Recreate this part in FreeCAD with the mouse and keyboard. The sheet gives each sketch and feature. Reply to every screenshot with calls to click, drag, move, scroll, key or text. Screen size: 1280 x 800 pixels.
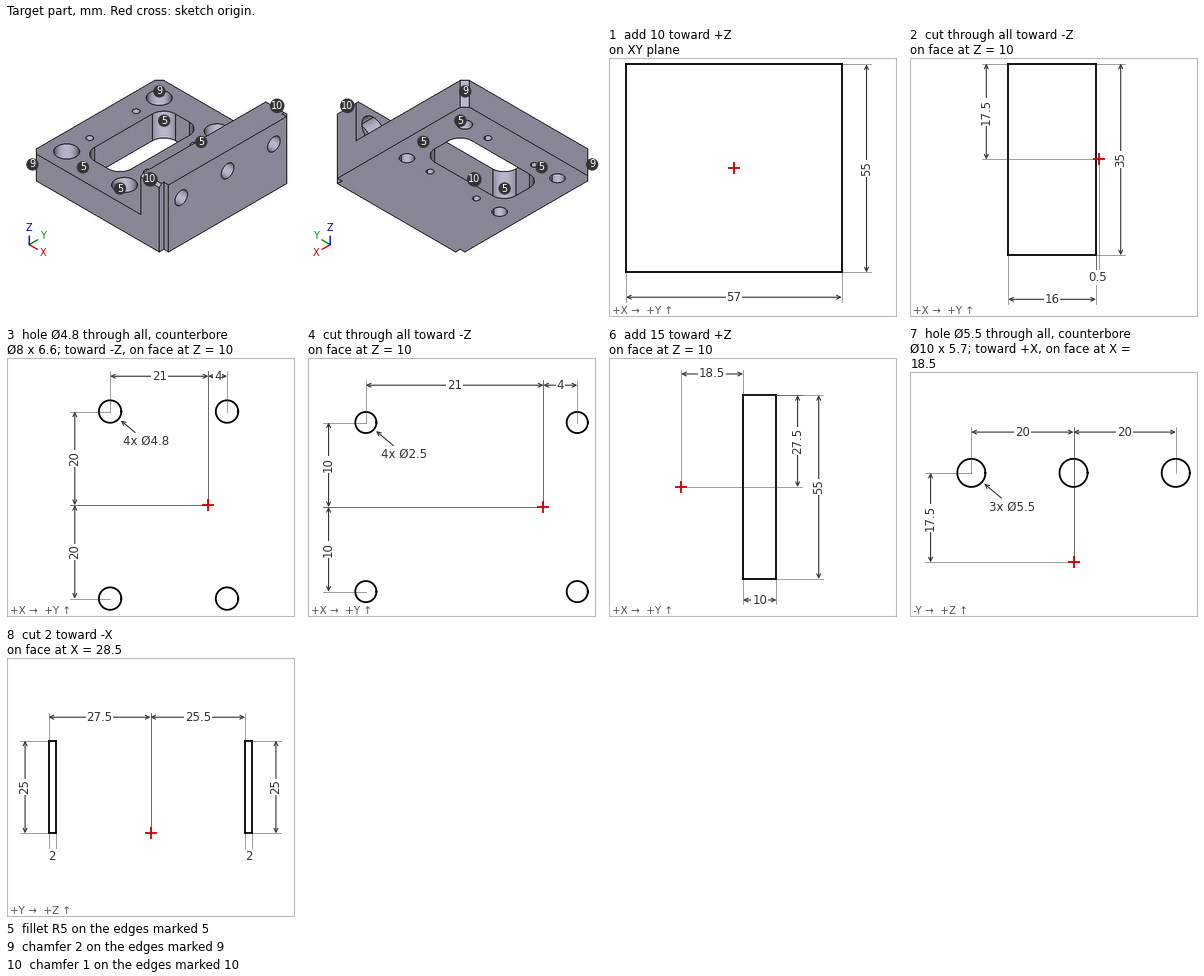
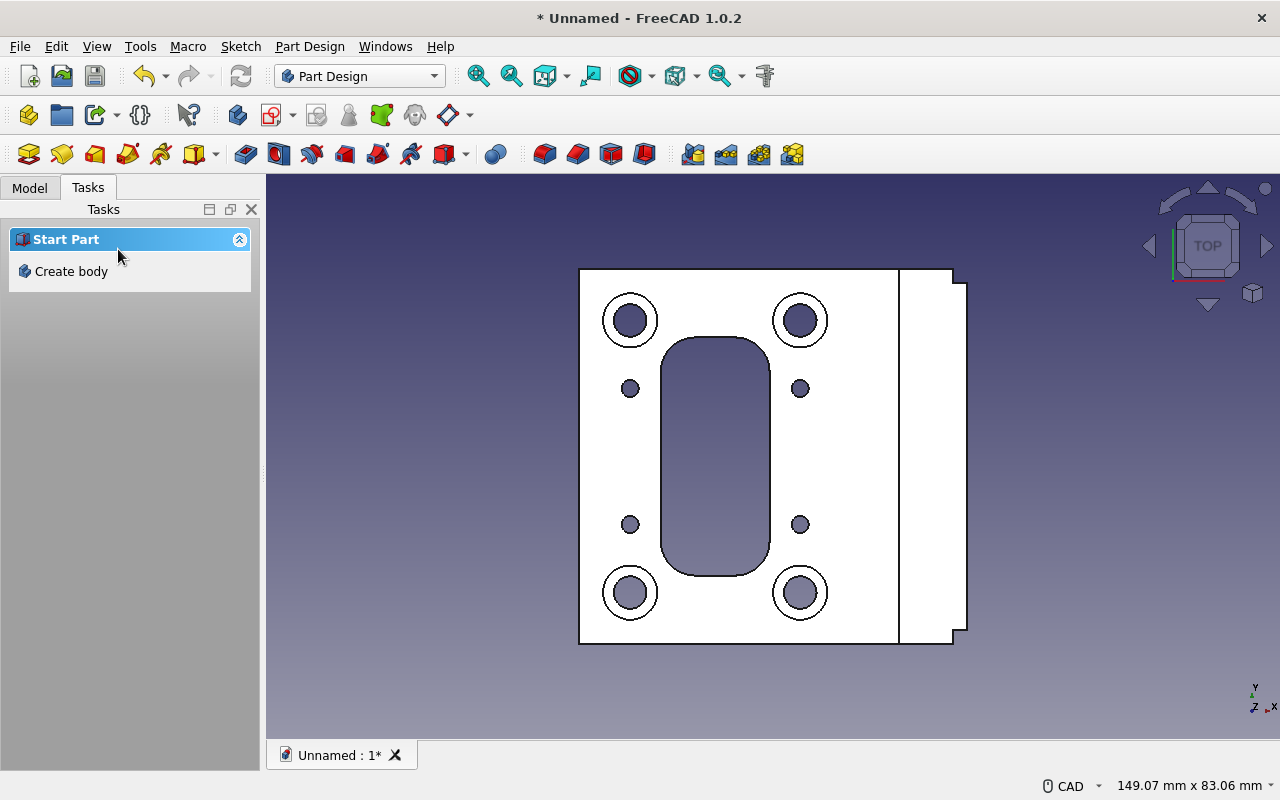
key(0)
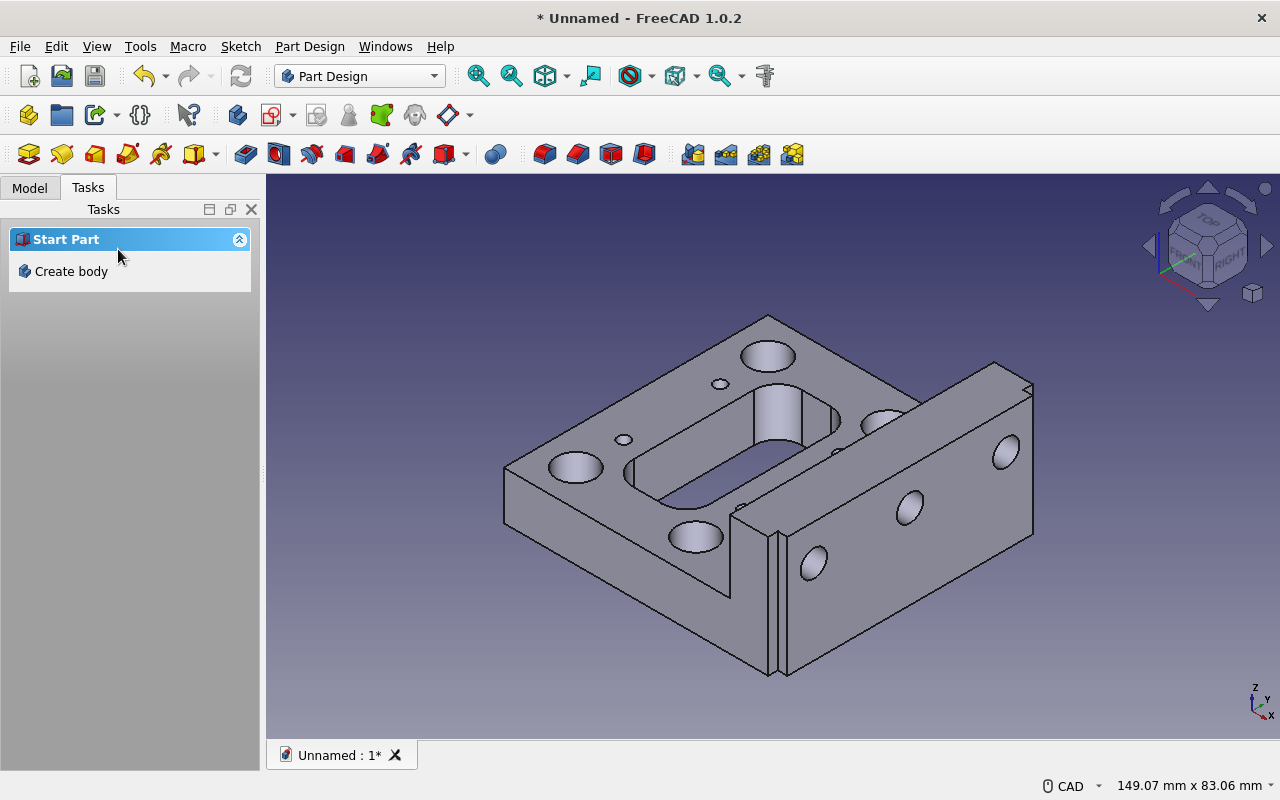
key(1)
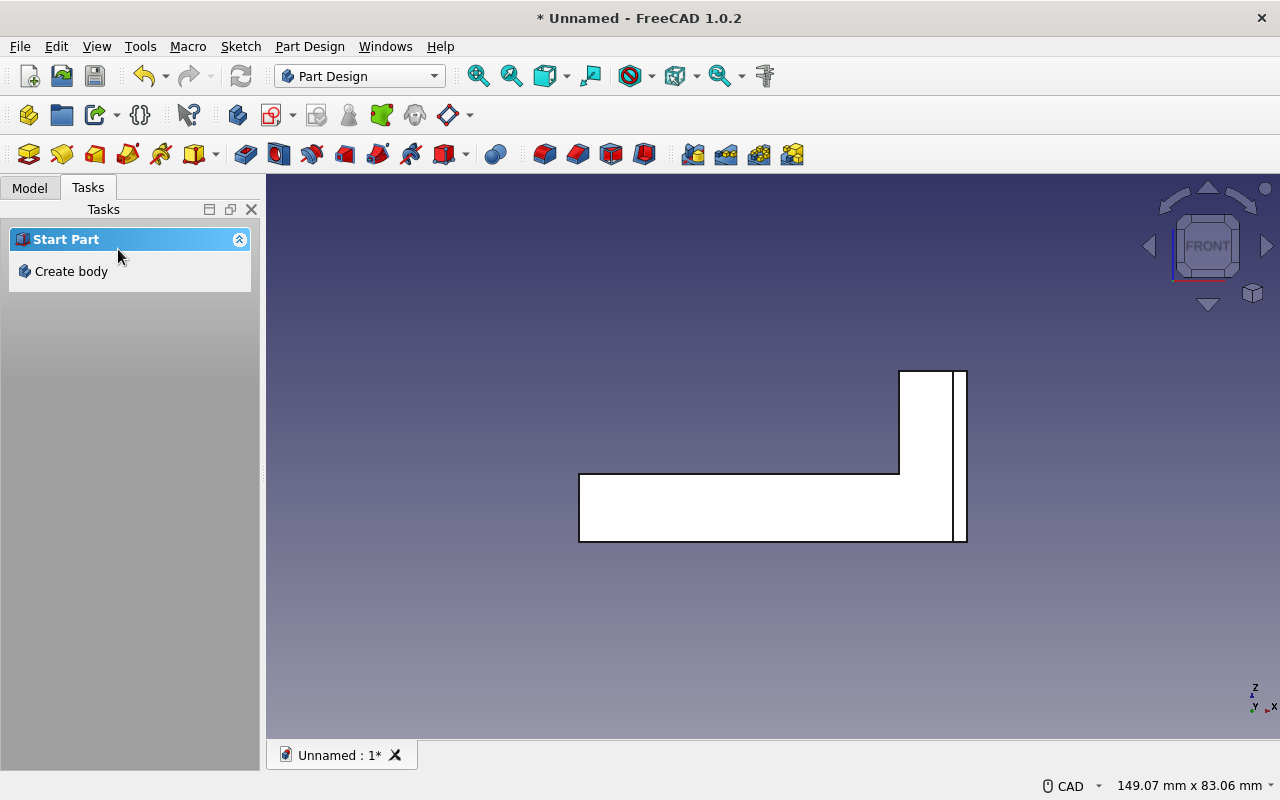
click(479, 76)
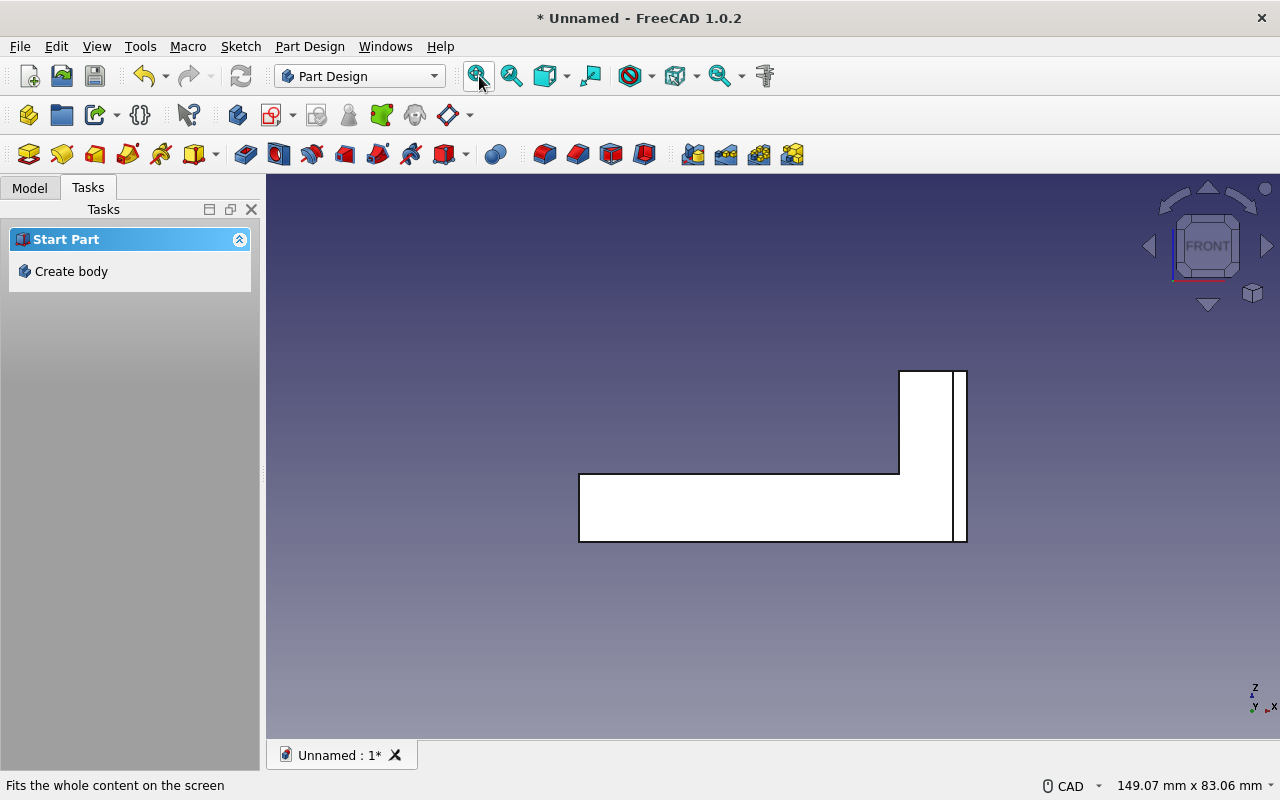
click(579, 507)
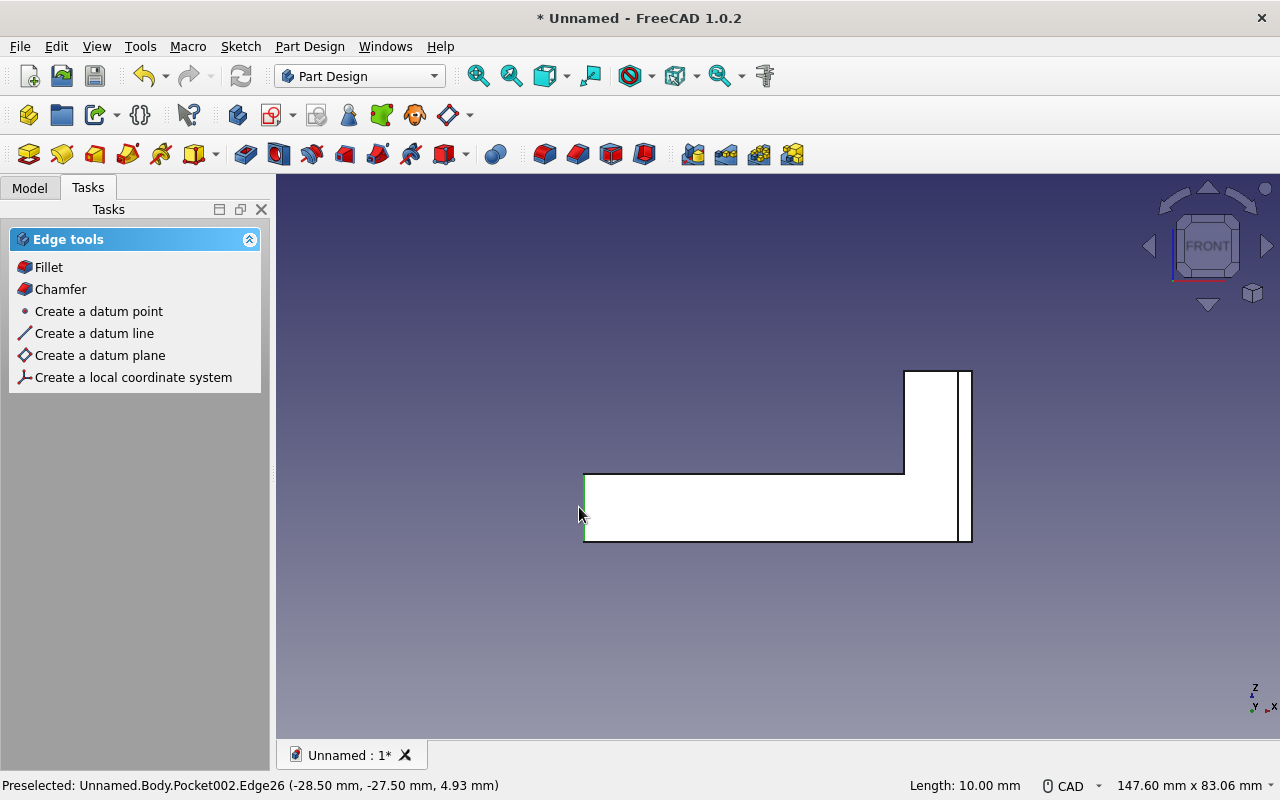
key(3)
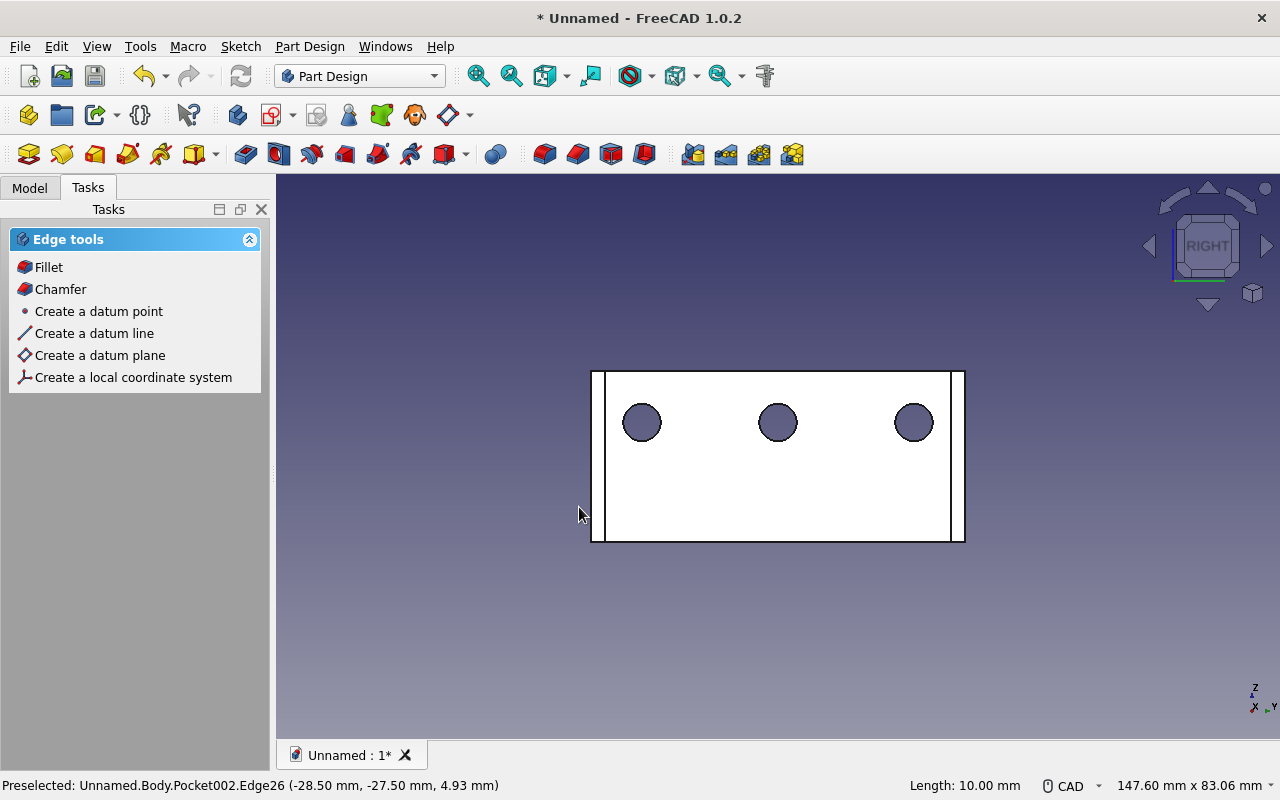
click(479, 76)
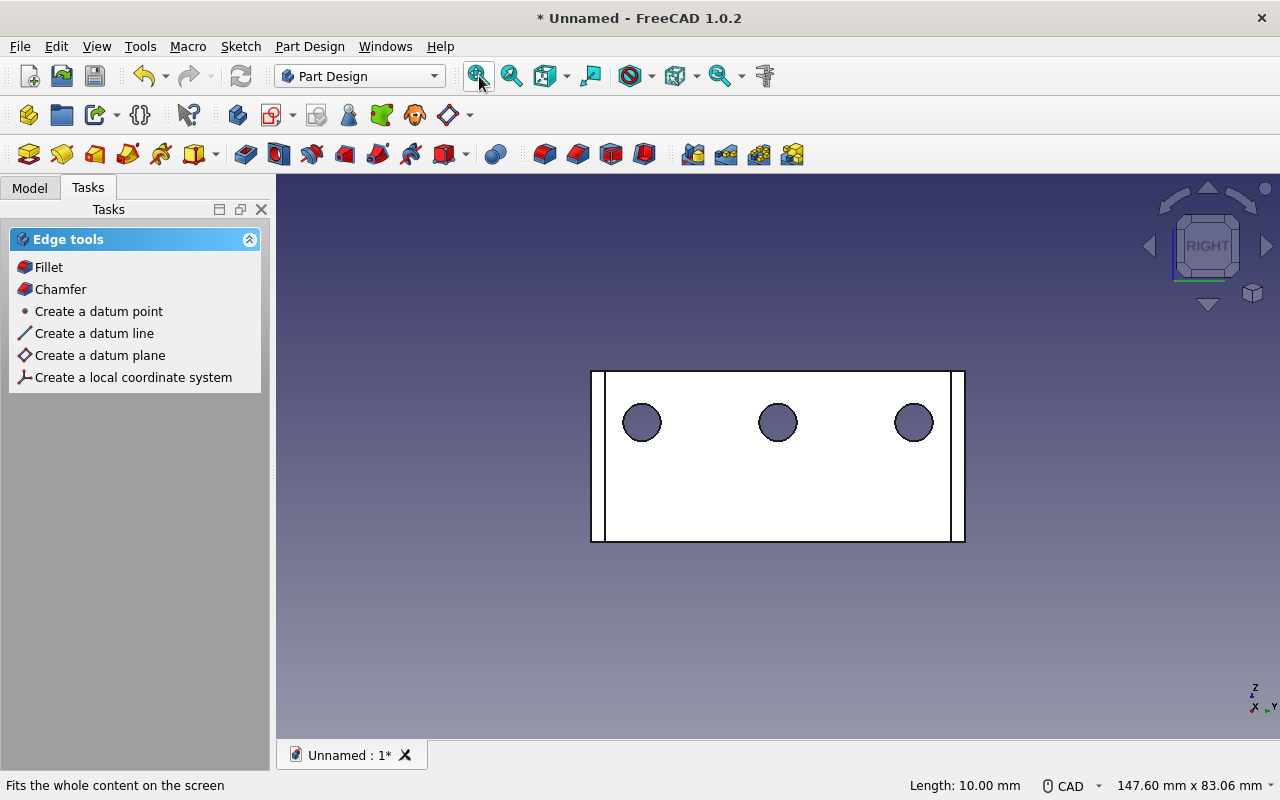
key(5)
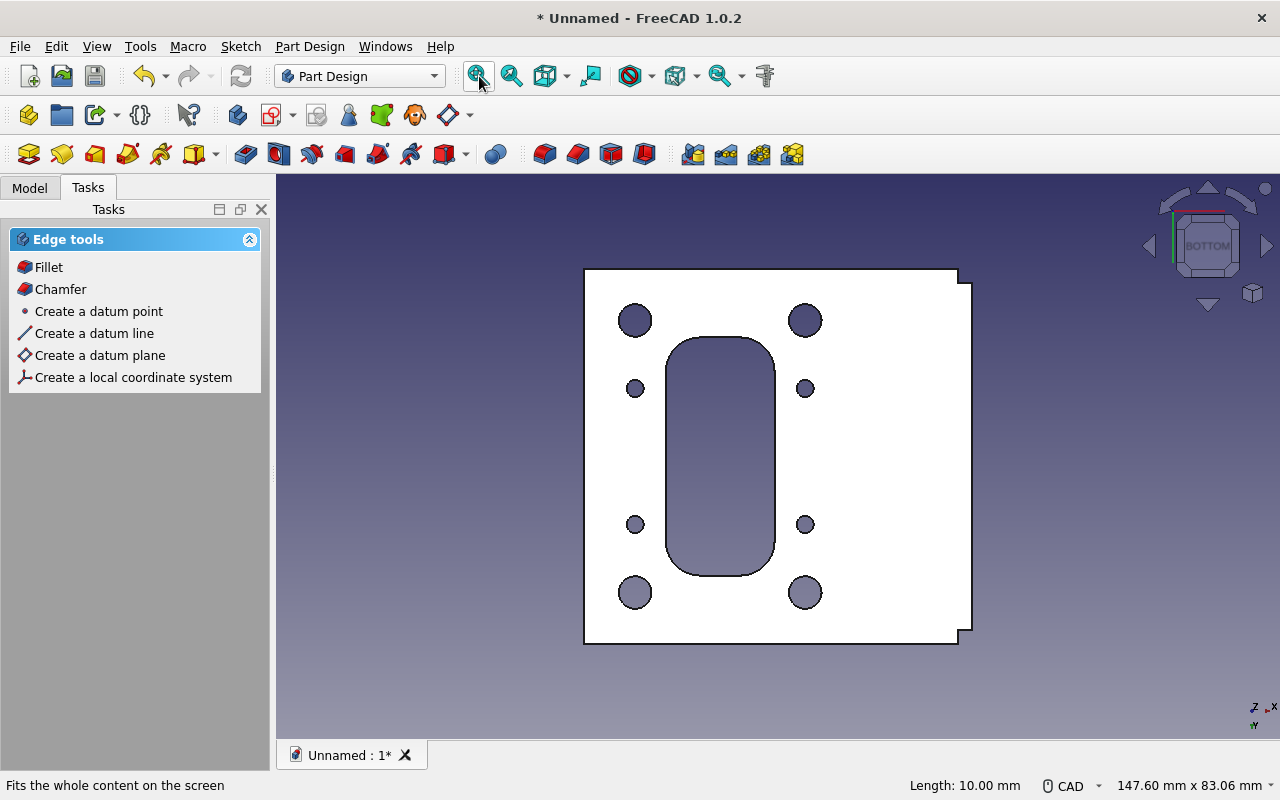
key(4)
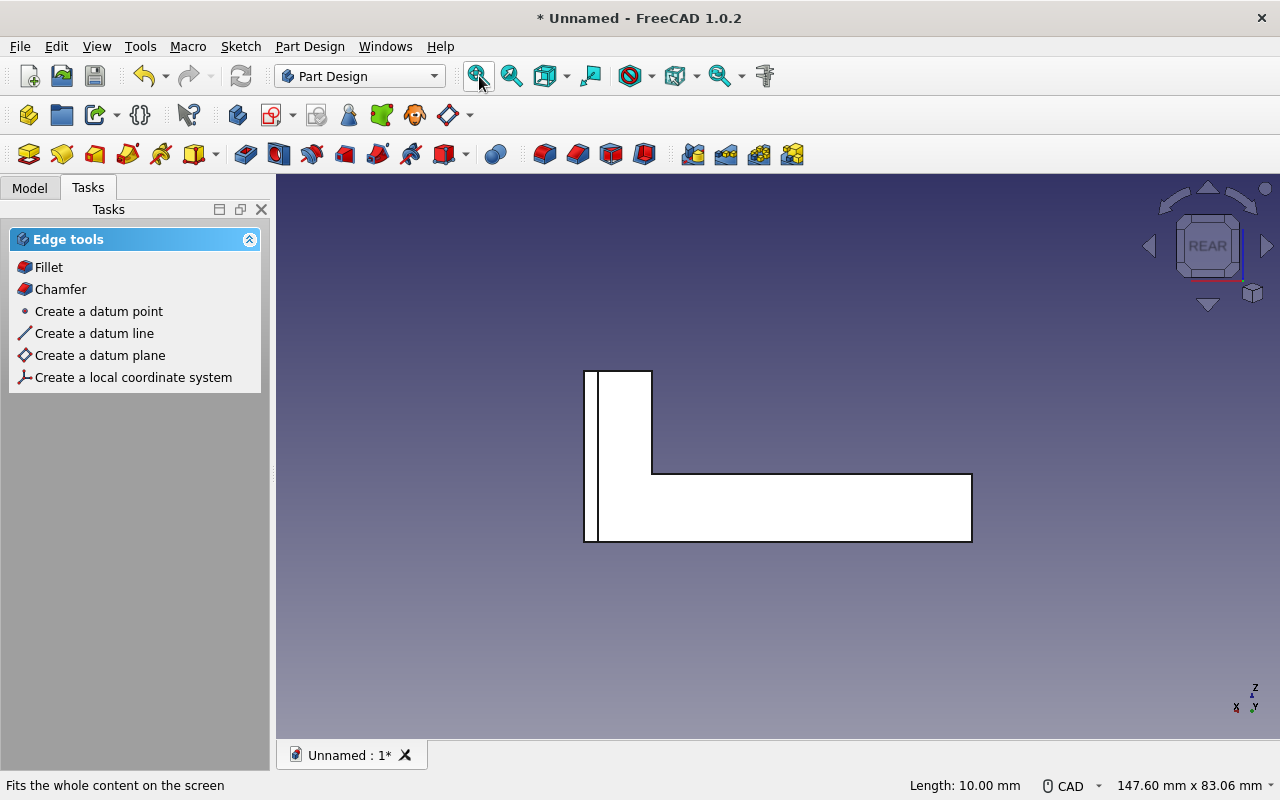
click(479, 76)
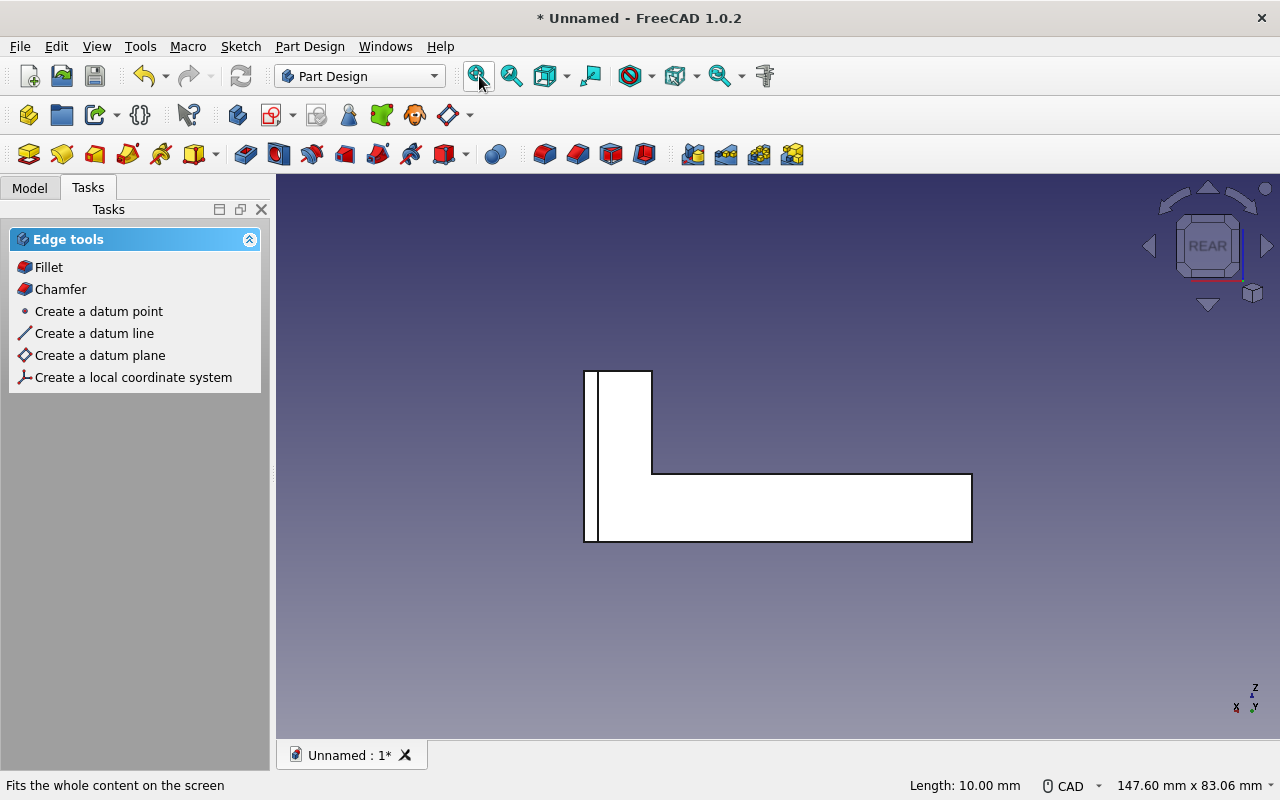
click(972, 507, ctrl)